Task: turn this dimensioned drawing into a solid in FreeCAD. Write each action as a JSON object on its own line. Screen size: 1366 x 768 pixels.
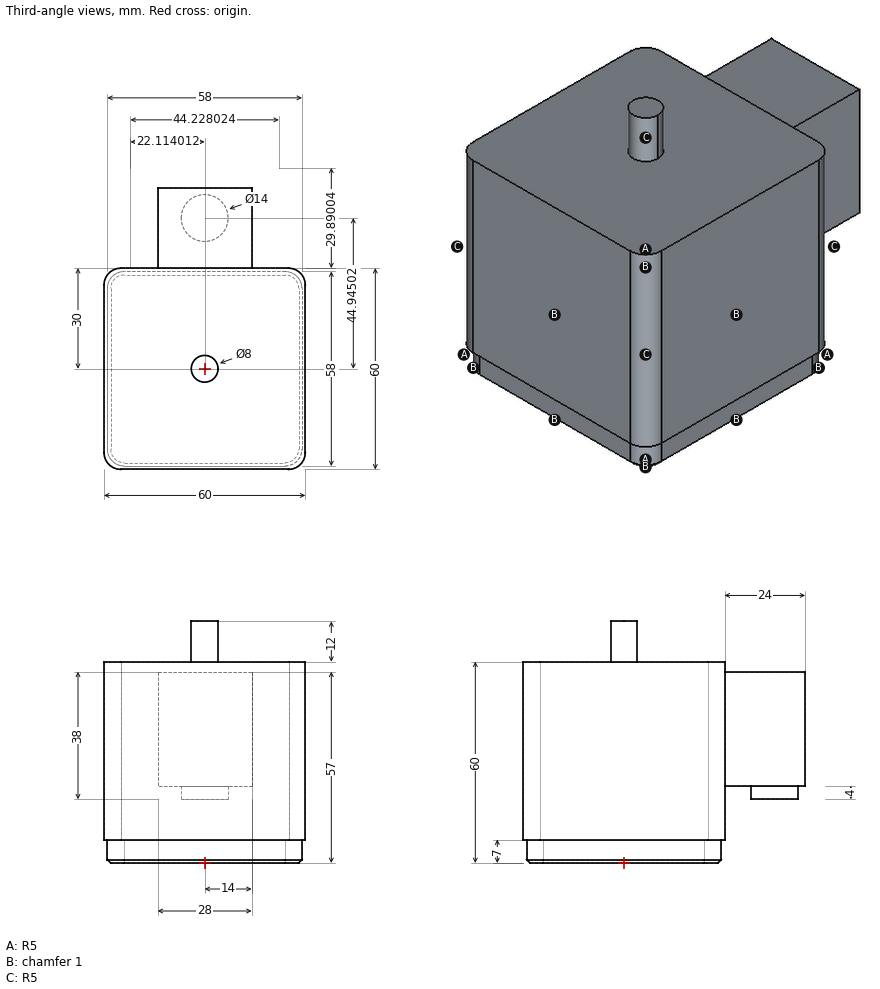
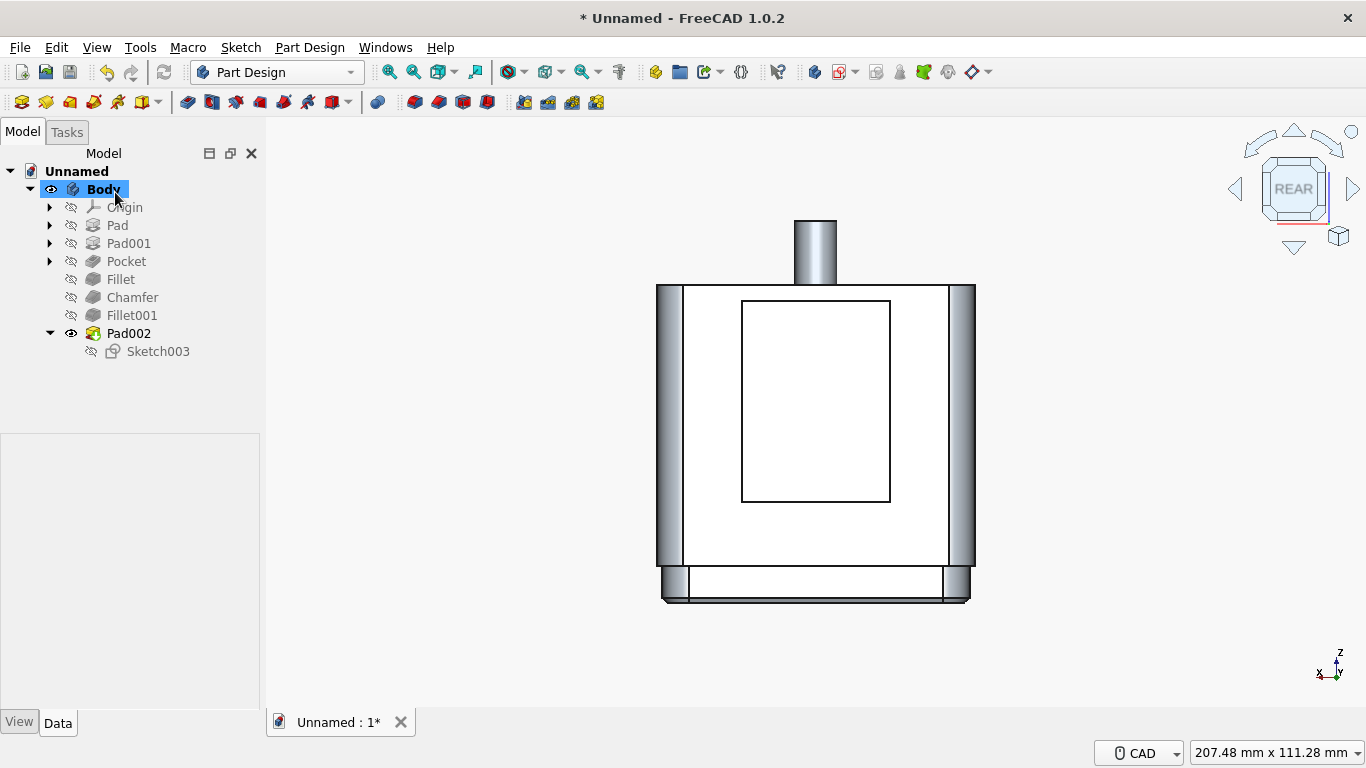
{"action": "key", "text": "5"}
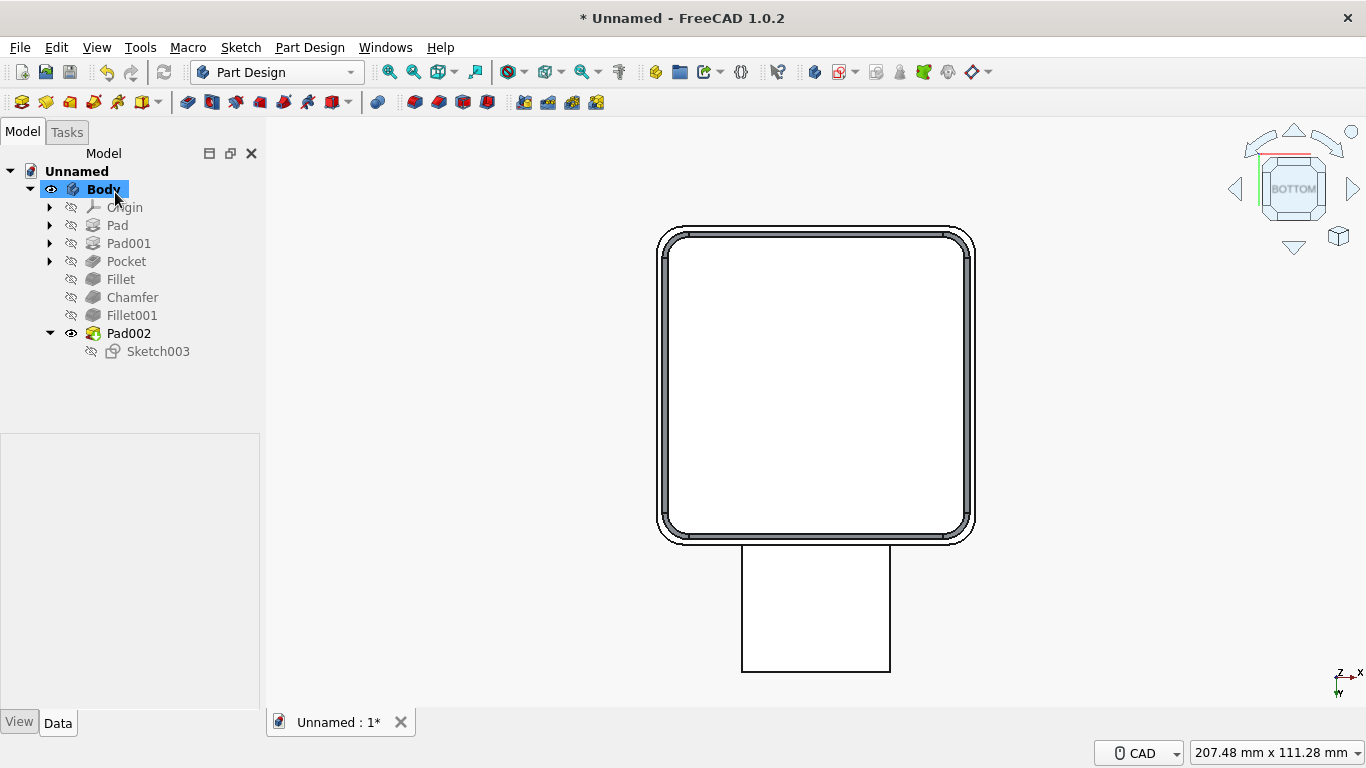
{"action": "left_click", "coordinate": [816, 607]}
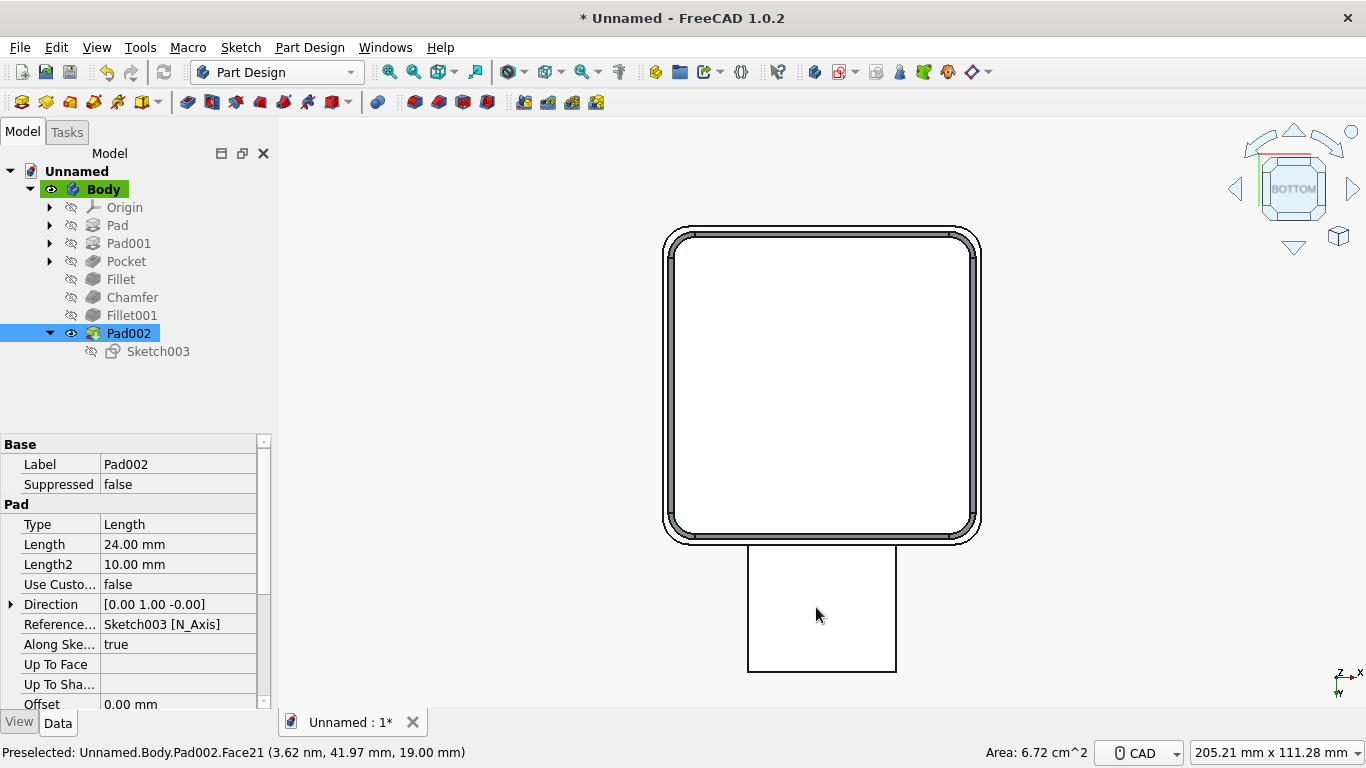
{"action": "left_click", "coordinate": [840, 72]}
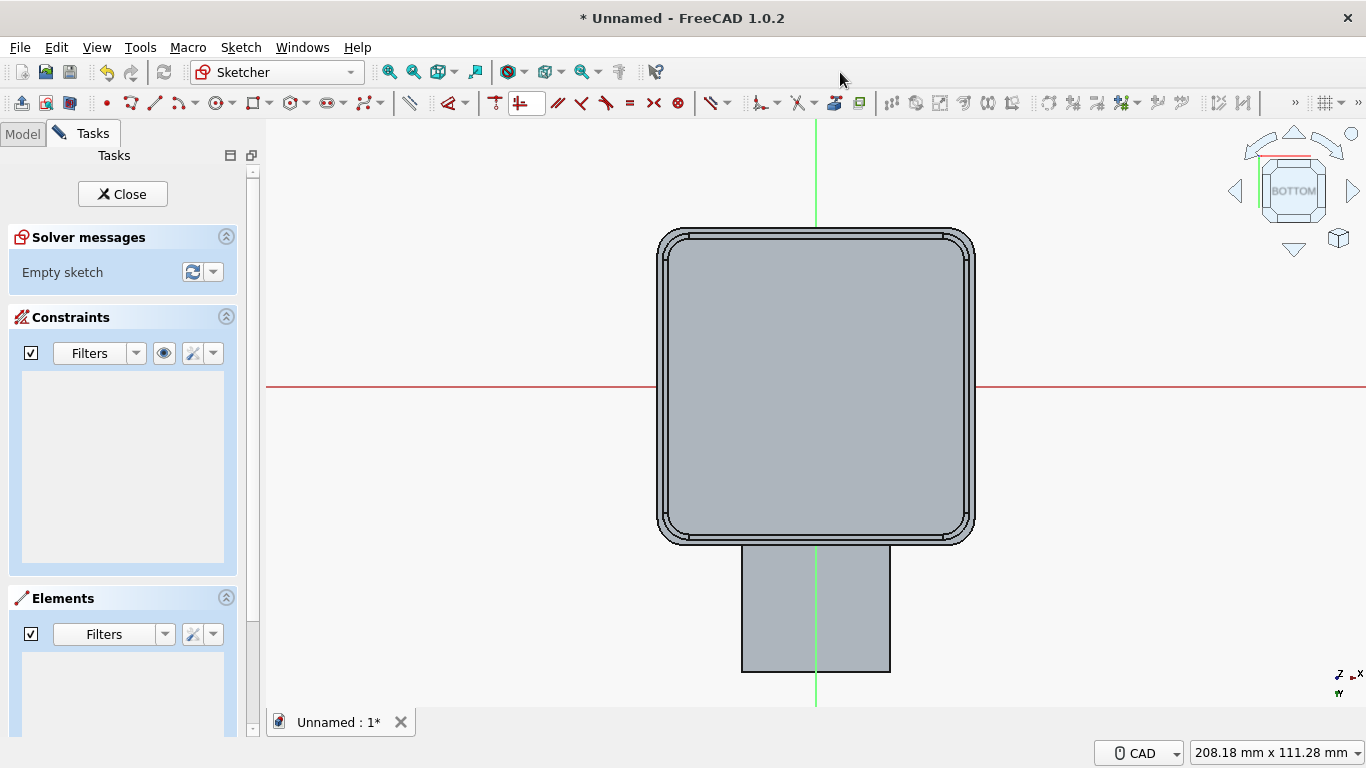
{"action": "left_click", "coordinate": [70, 104]}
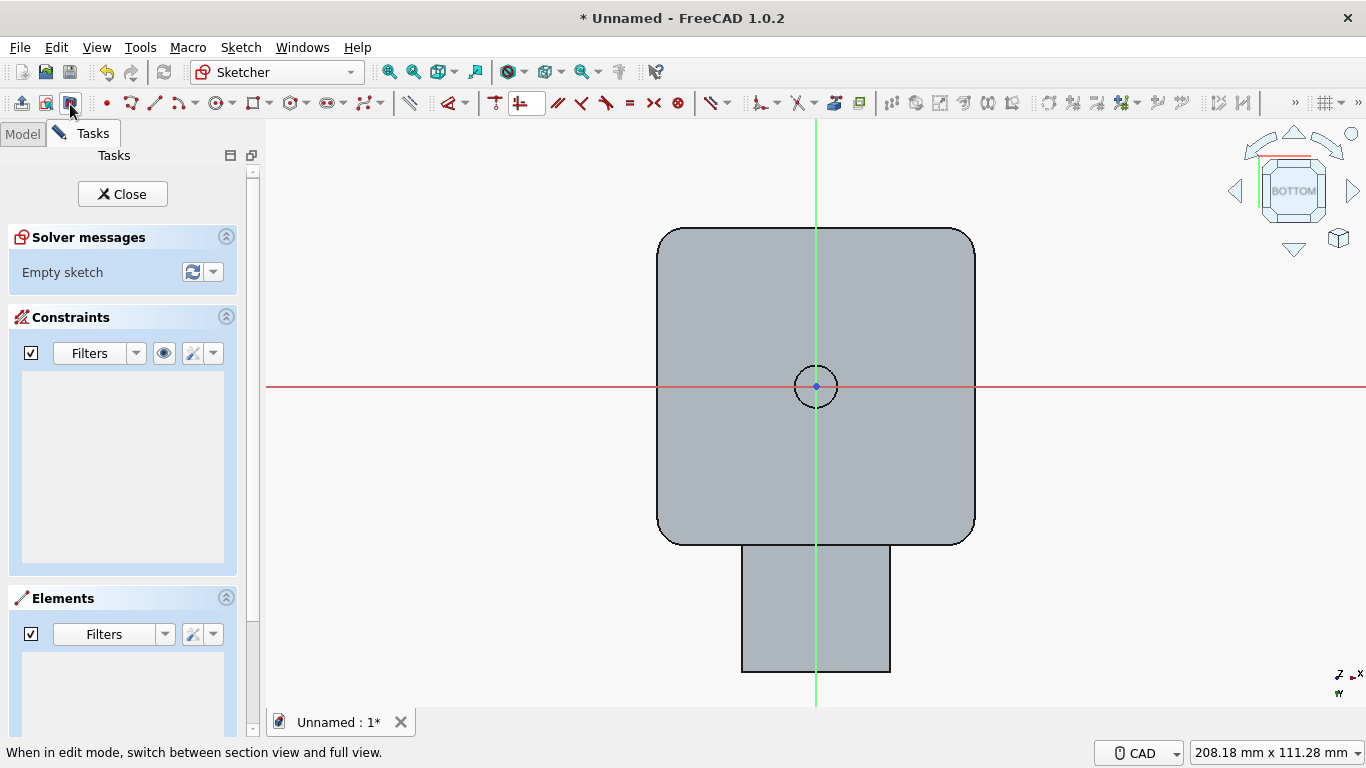
{"action": "scroll", "coordinate": [438, 147], "scroll_direction": "down", "scroll_amount": 1}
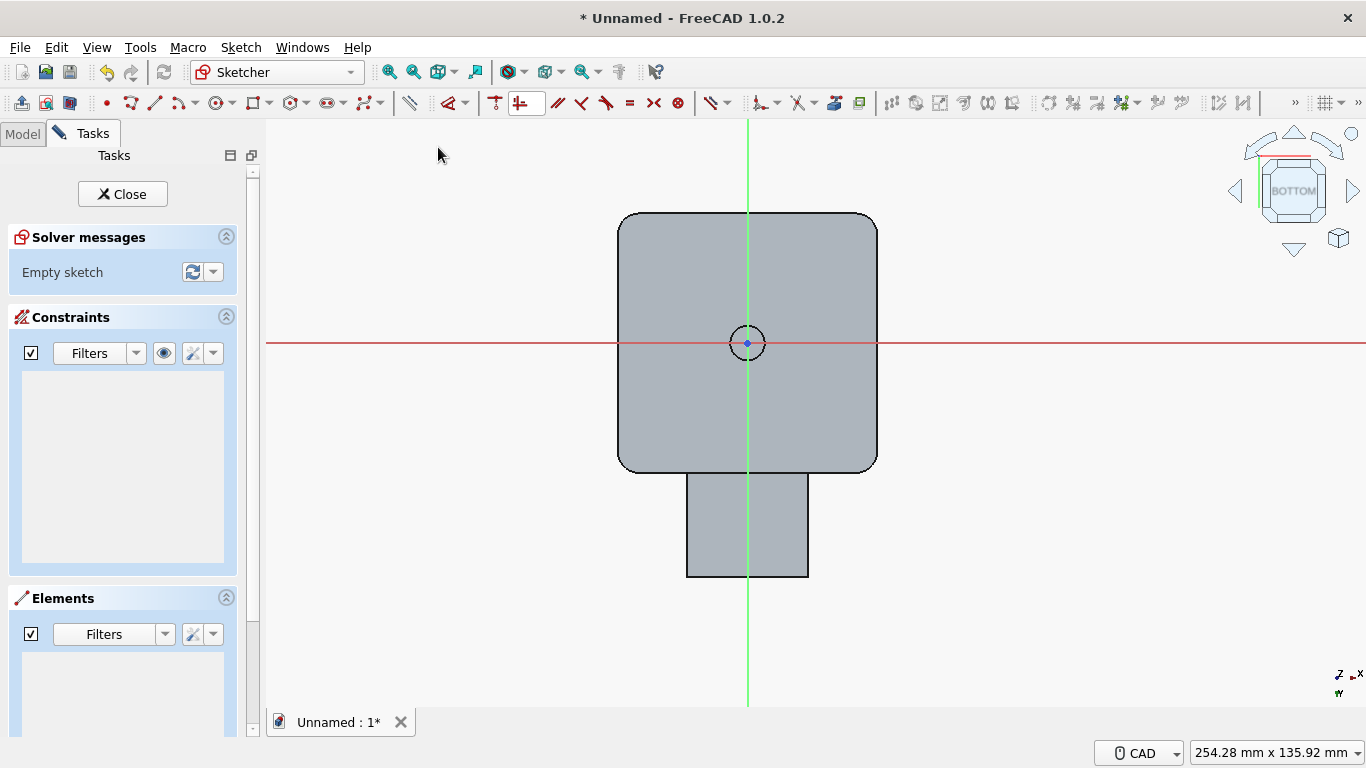
{"action": "scroll", "coordinate": [748, 594], "scroll_direction": "up", "scroll_amount": 2}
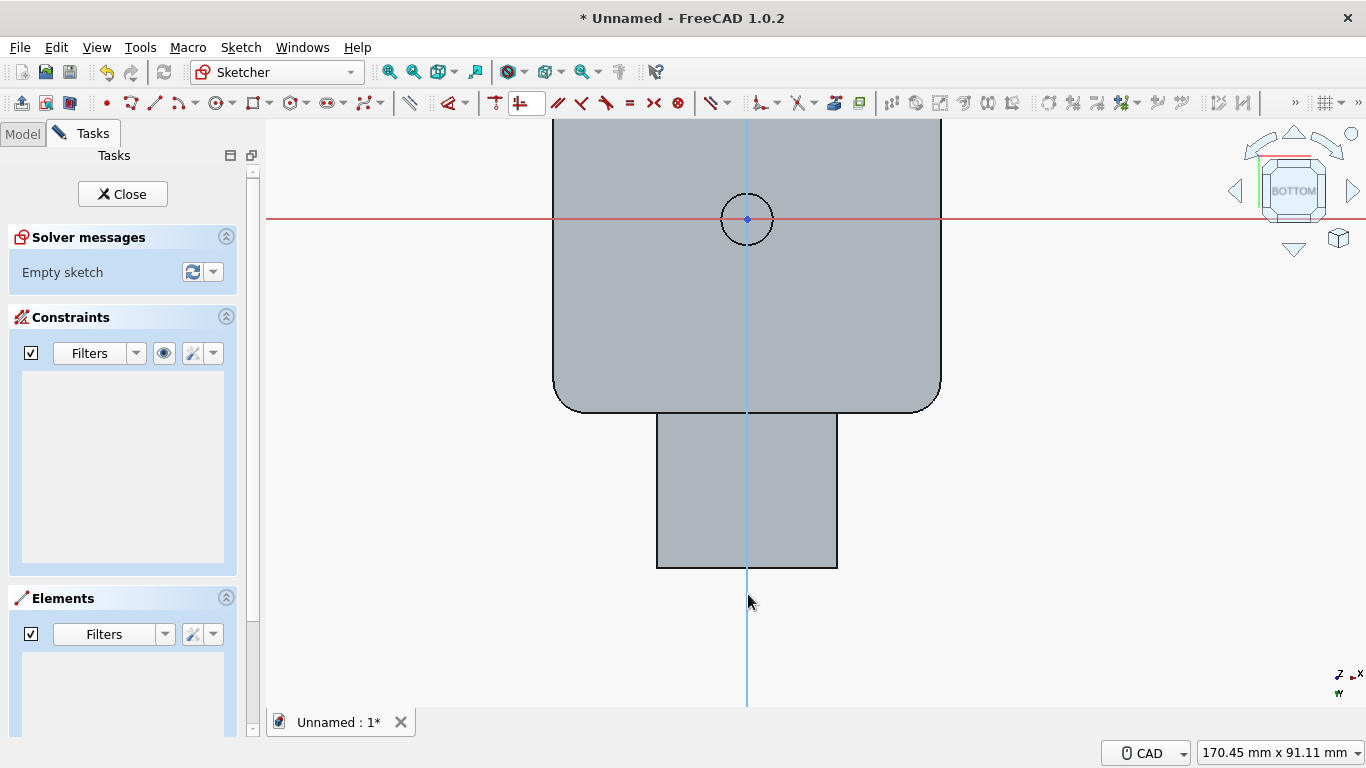
{"action": "key", "text": "g r"}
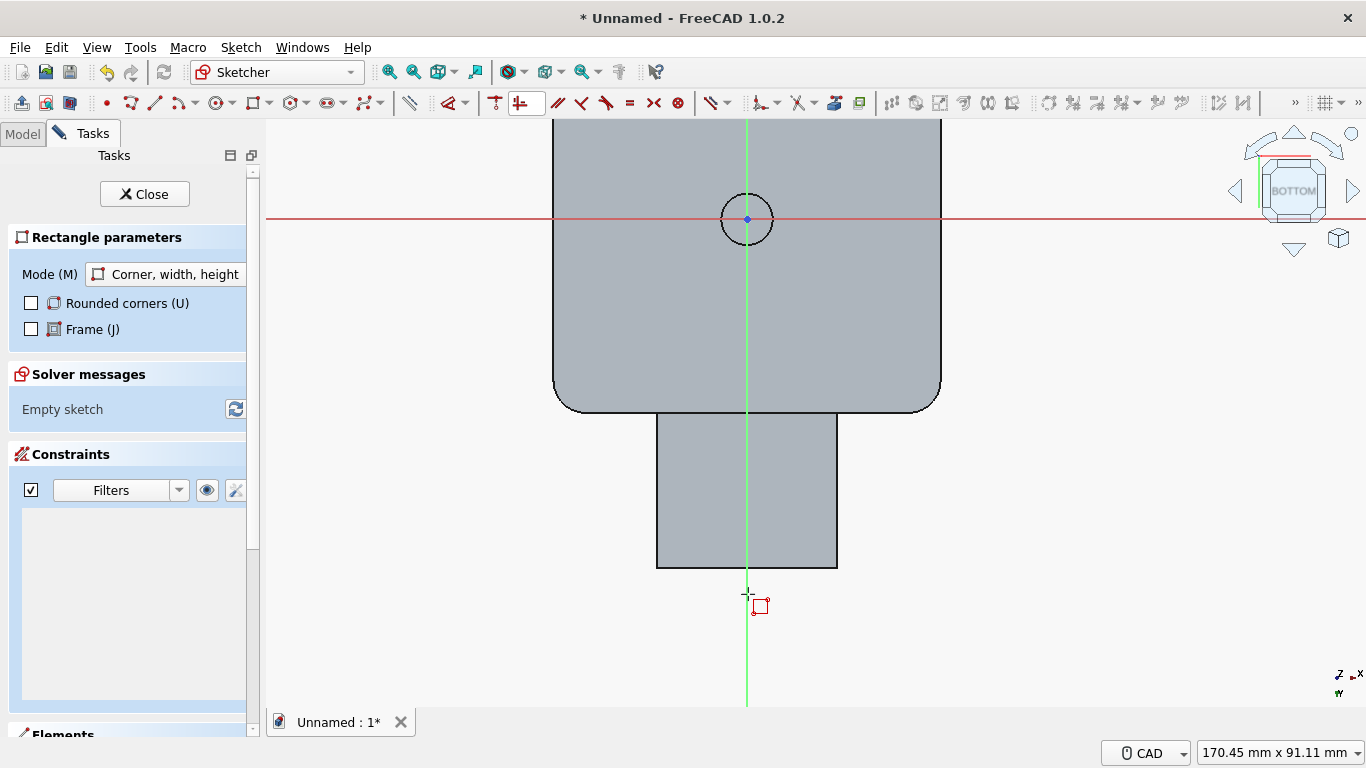
{"action": "left_click", "coordinate": [604, 413]}
{"action": "mouse_move", "coordinate": [890, 606]}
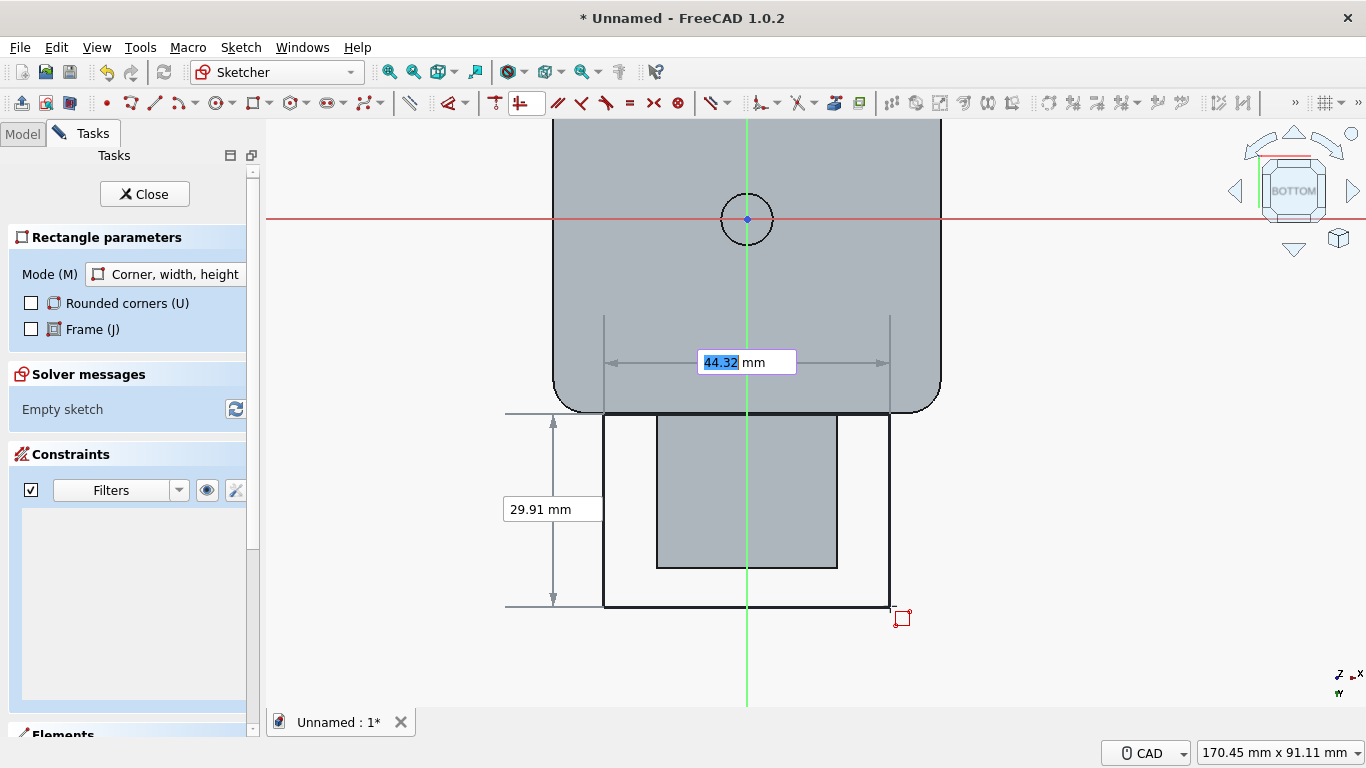
{"action": "type", "text": "44.228024"}
{"action": "key", "text": "Tab"}
{"action": "type", "text": "29.89004"}
{"action": "key", "text": "Return"}